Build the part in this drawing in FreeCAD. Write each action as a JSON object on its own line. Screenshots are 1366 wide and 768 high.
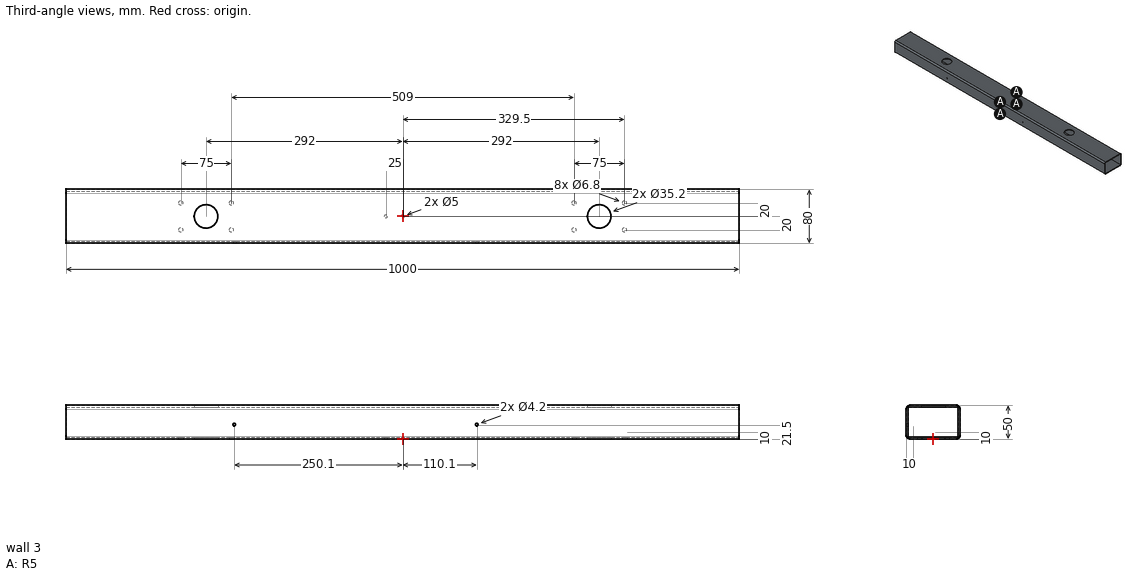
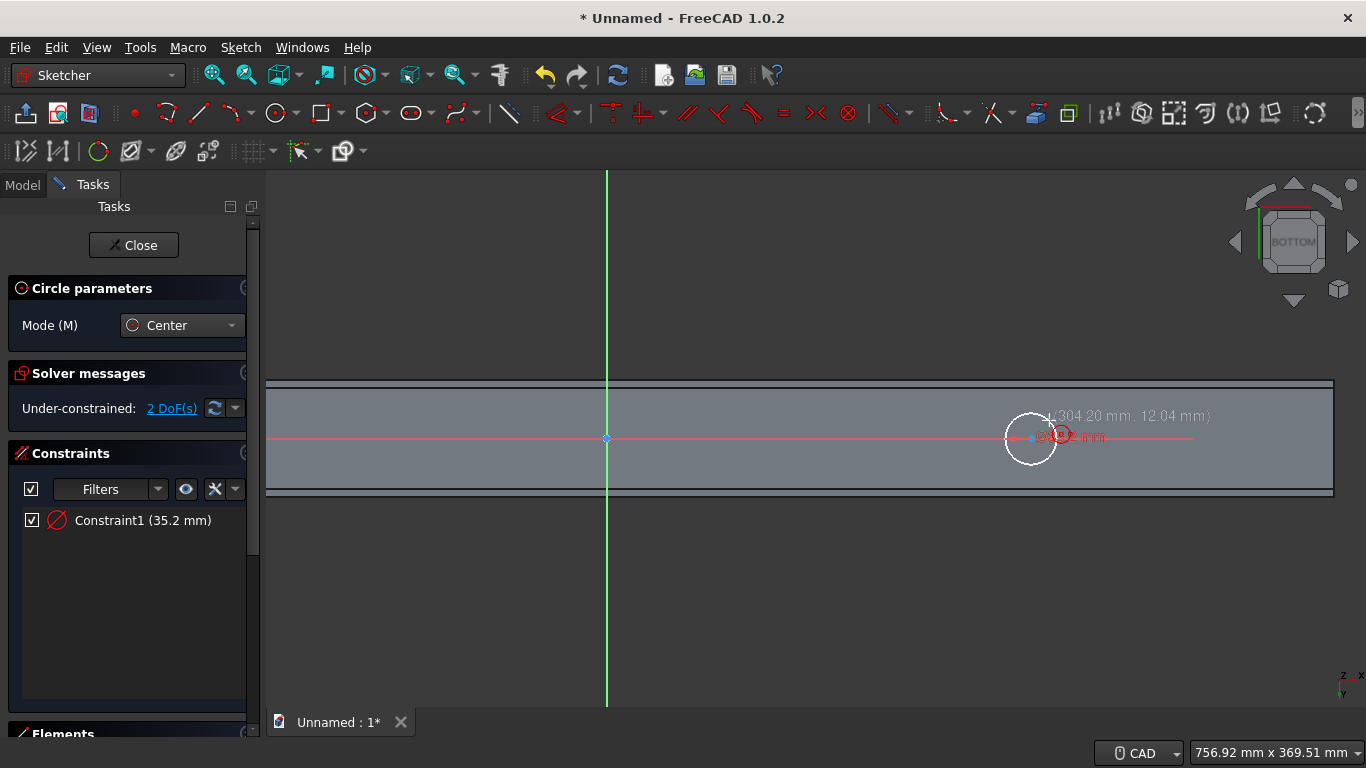
{"action": "scroll", "coordinate": [1033, 438], "scroll_direction": "down", "scroll_amount": 2}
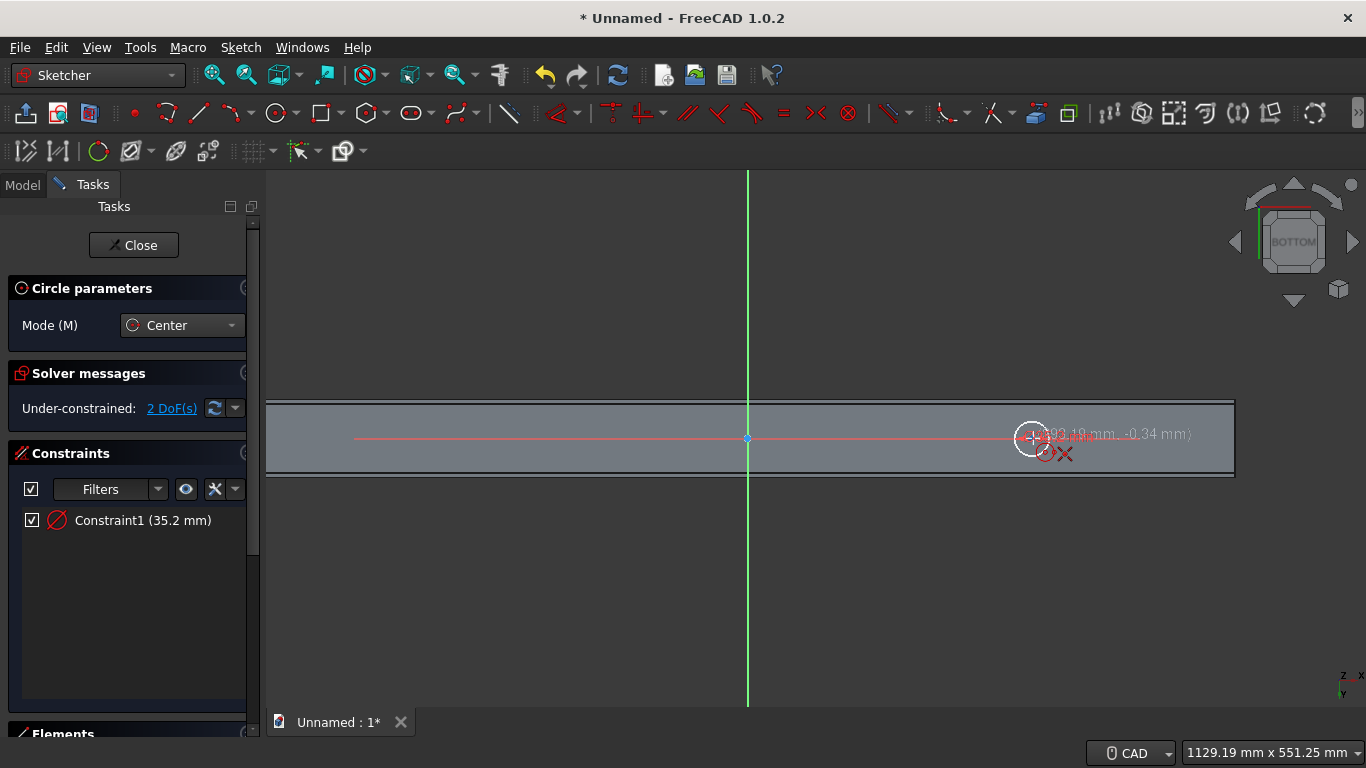
{"action": "scroll", "coordinate": [463, 438], "scroll_direction": "up", "scroll_amount": 2}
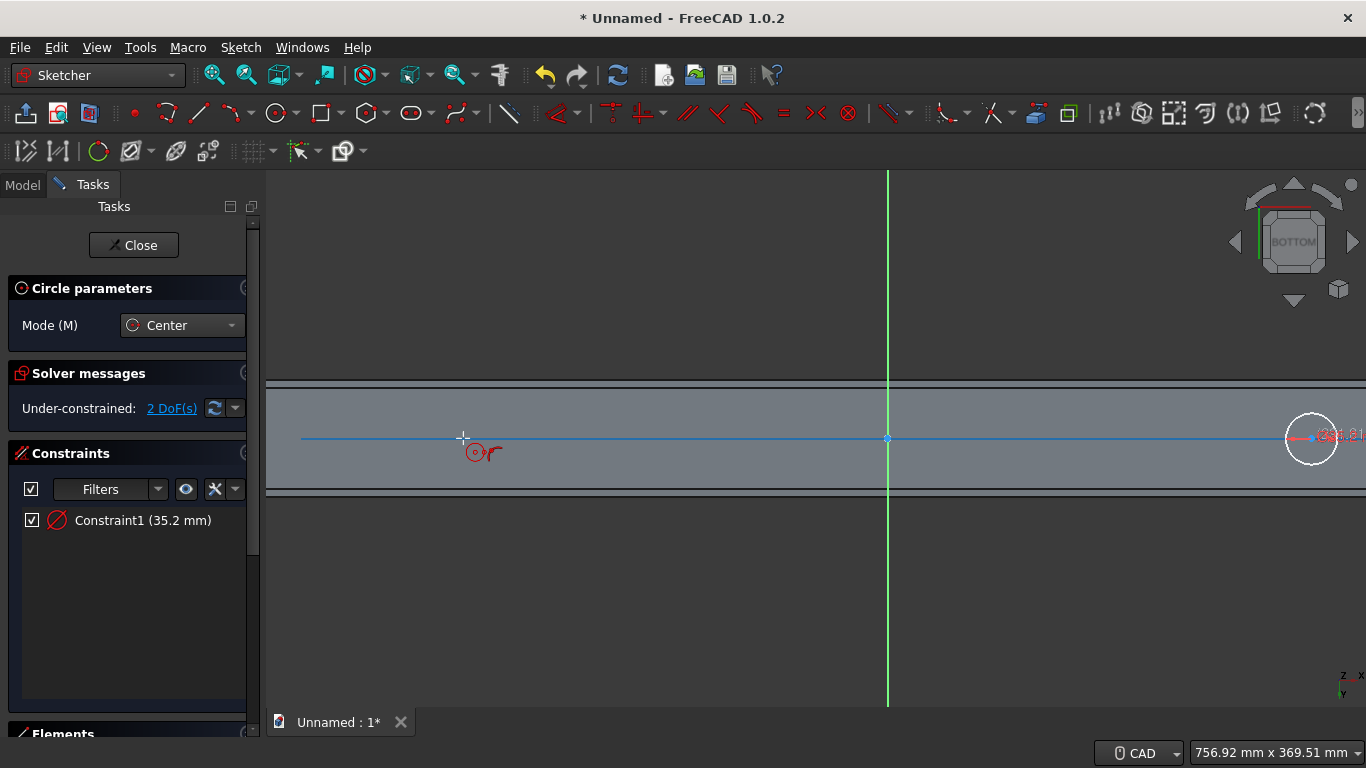
{"action": "left_click", "coordinate": [463, 438]}
{"action": "mouse_move", "coordinate": [481, 420]}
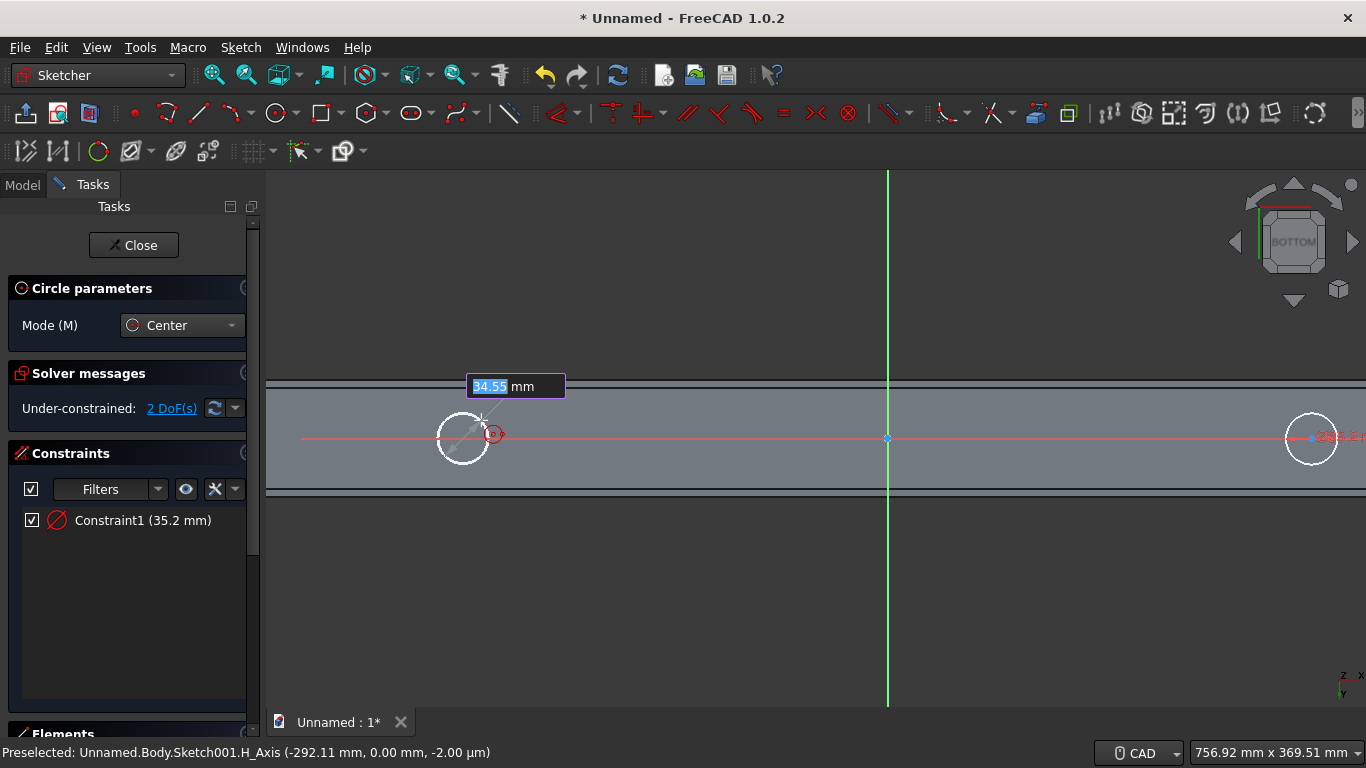
{"action": "type", "text": "35.2"}
{"action": "key", "text": "Return"}
{"action": "key", "text": "Escape"}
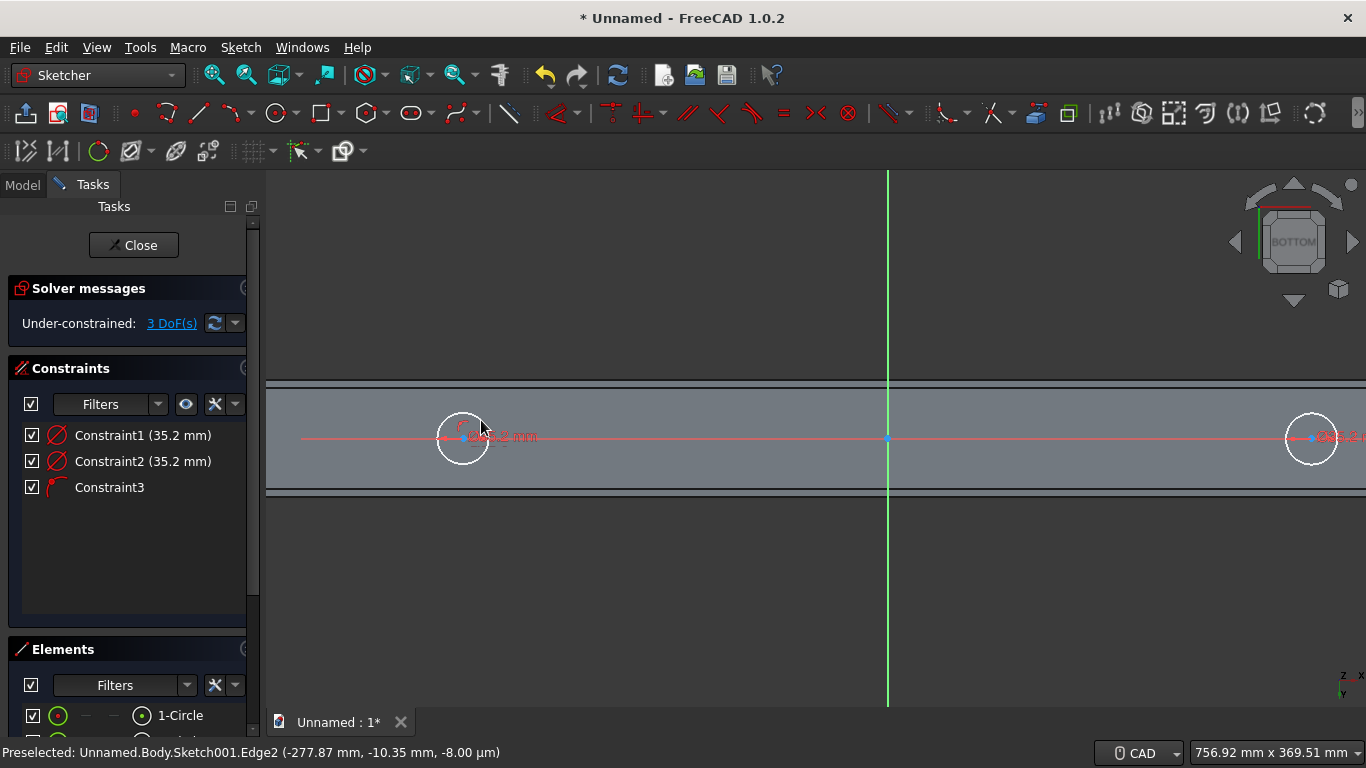
{"action": "scroll", "coordinate": [463, 438], "scroll_direction": "down", "scroll_amount": 2}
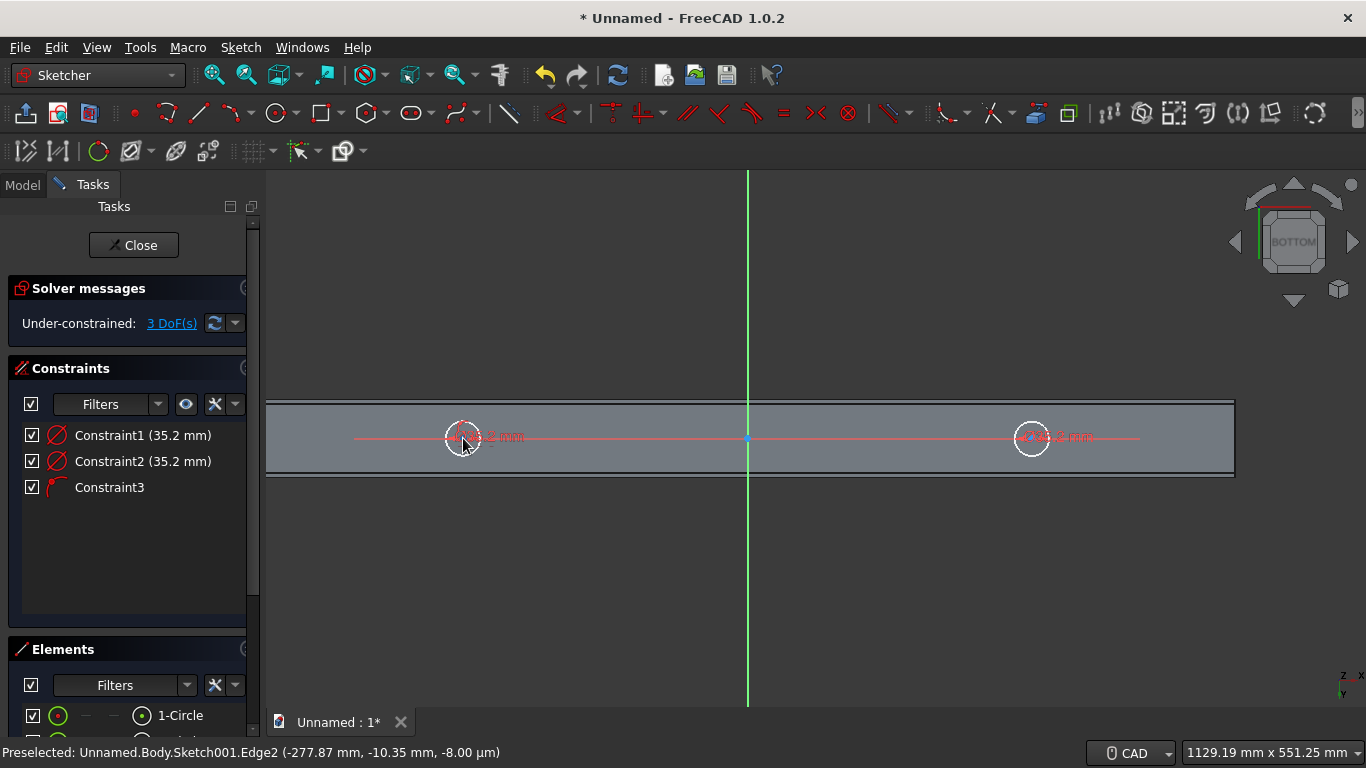
{"action": "left_click", "coordinate": [1032, 439]}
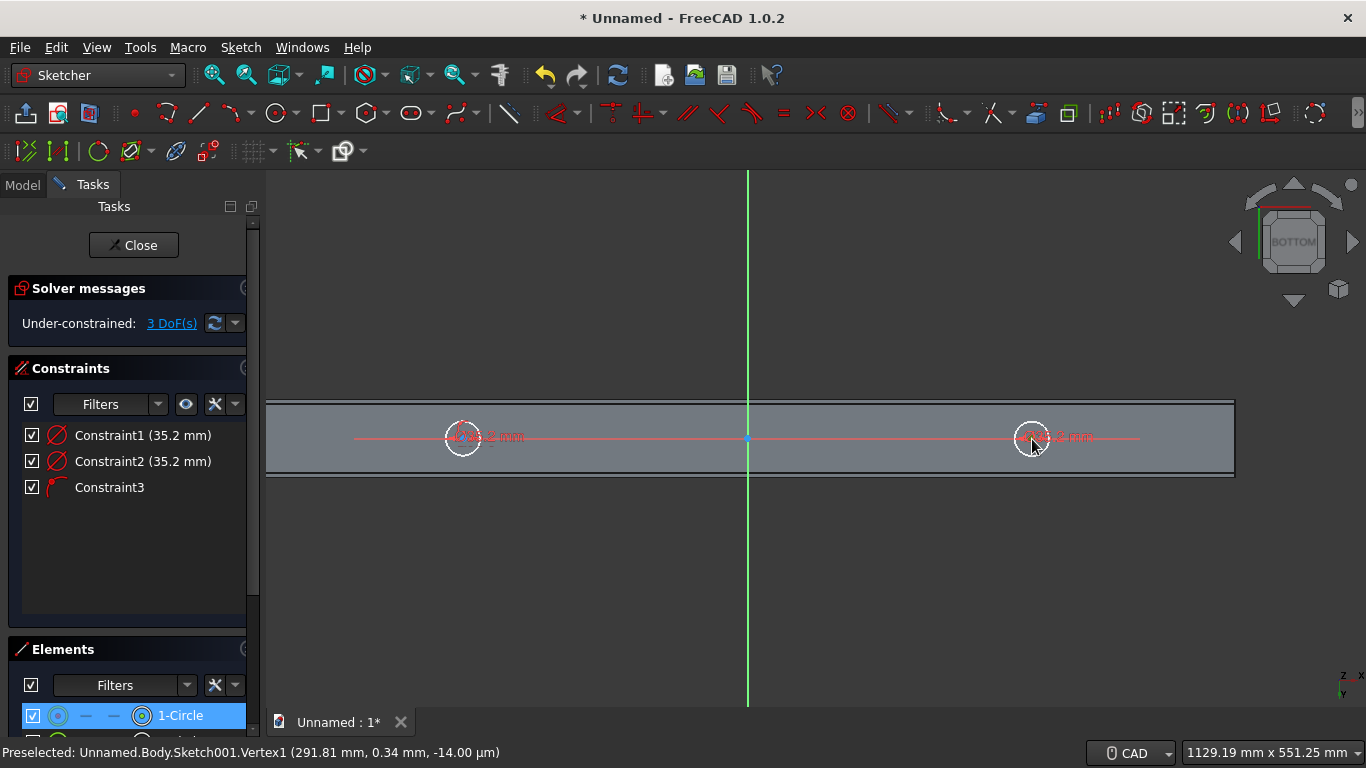
{"action": "left_click", "coordinate": [359, 438]}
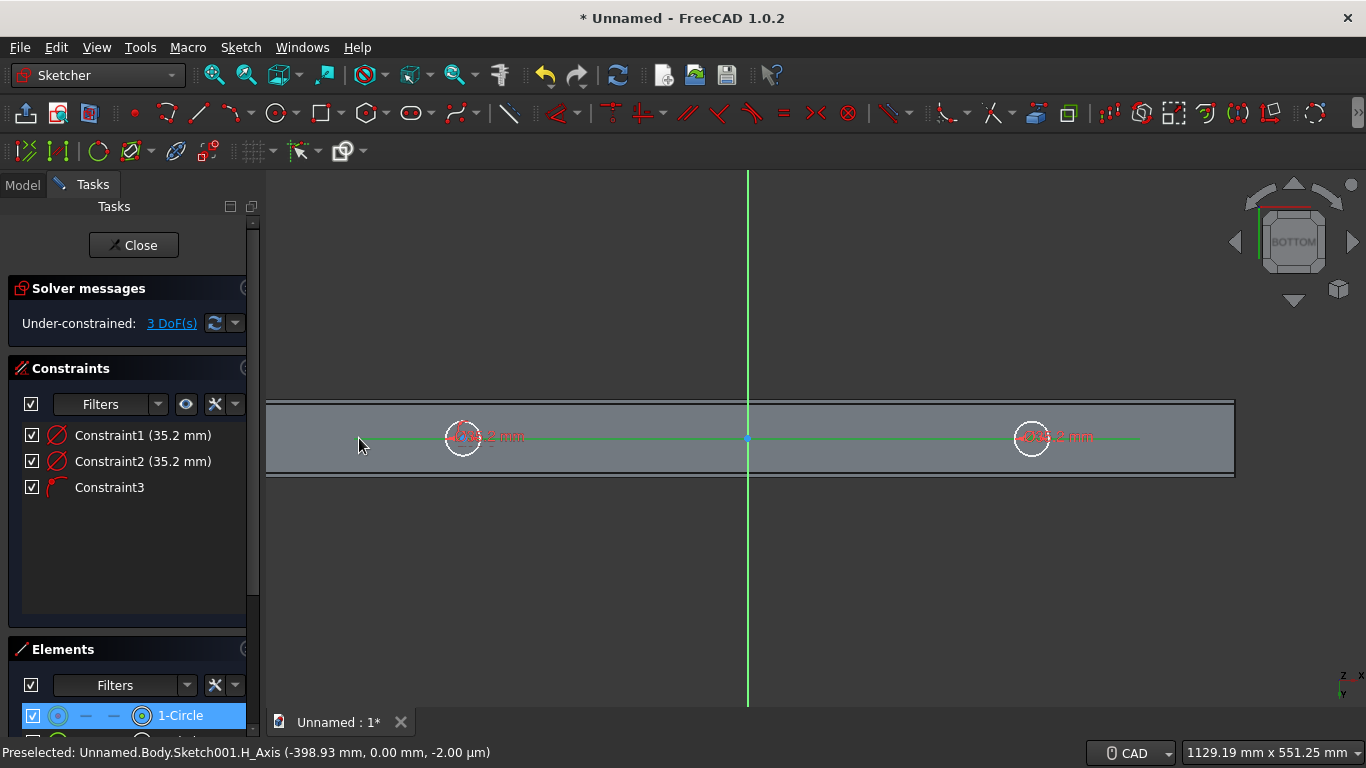
{"action": "key", "text": "c"}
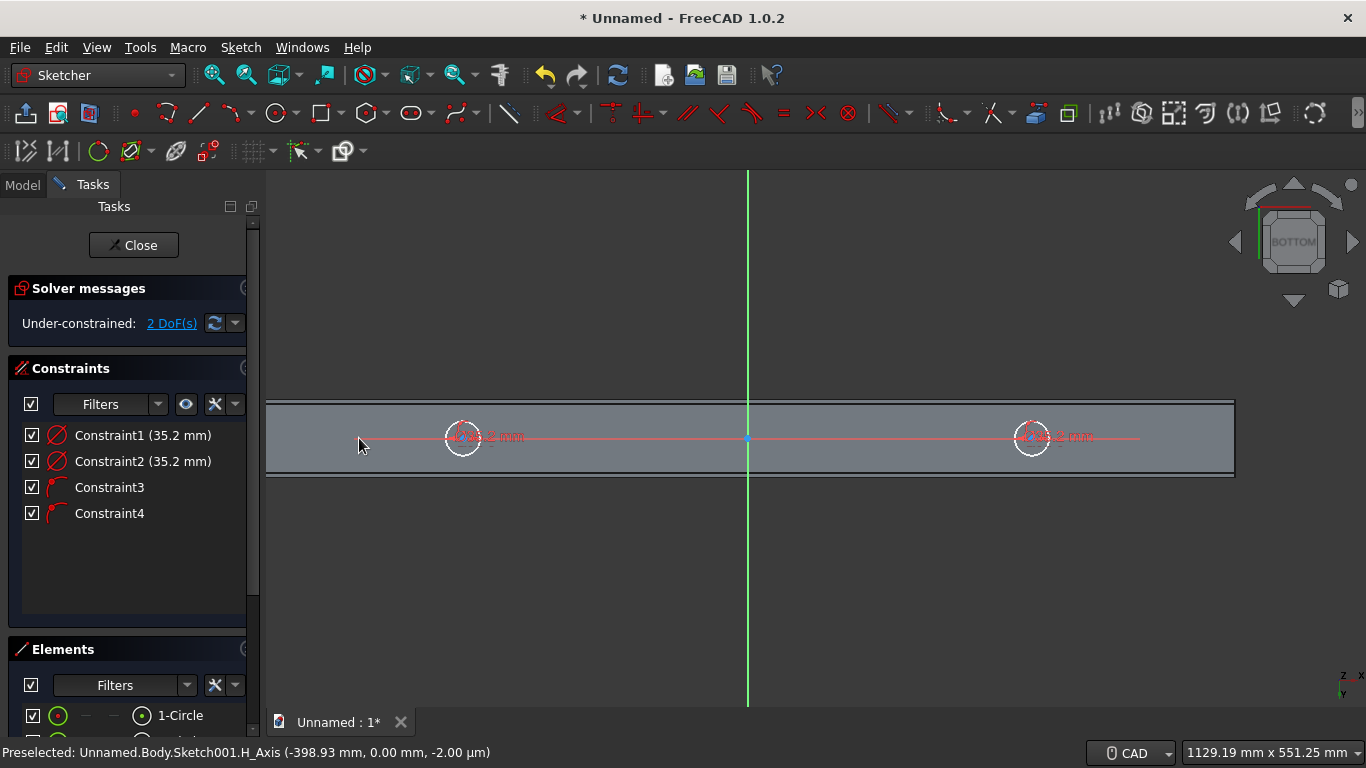
{"action": "left_click", "coordinate": [1032, 438]}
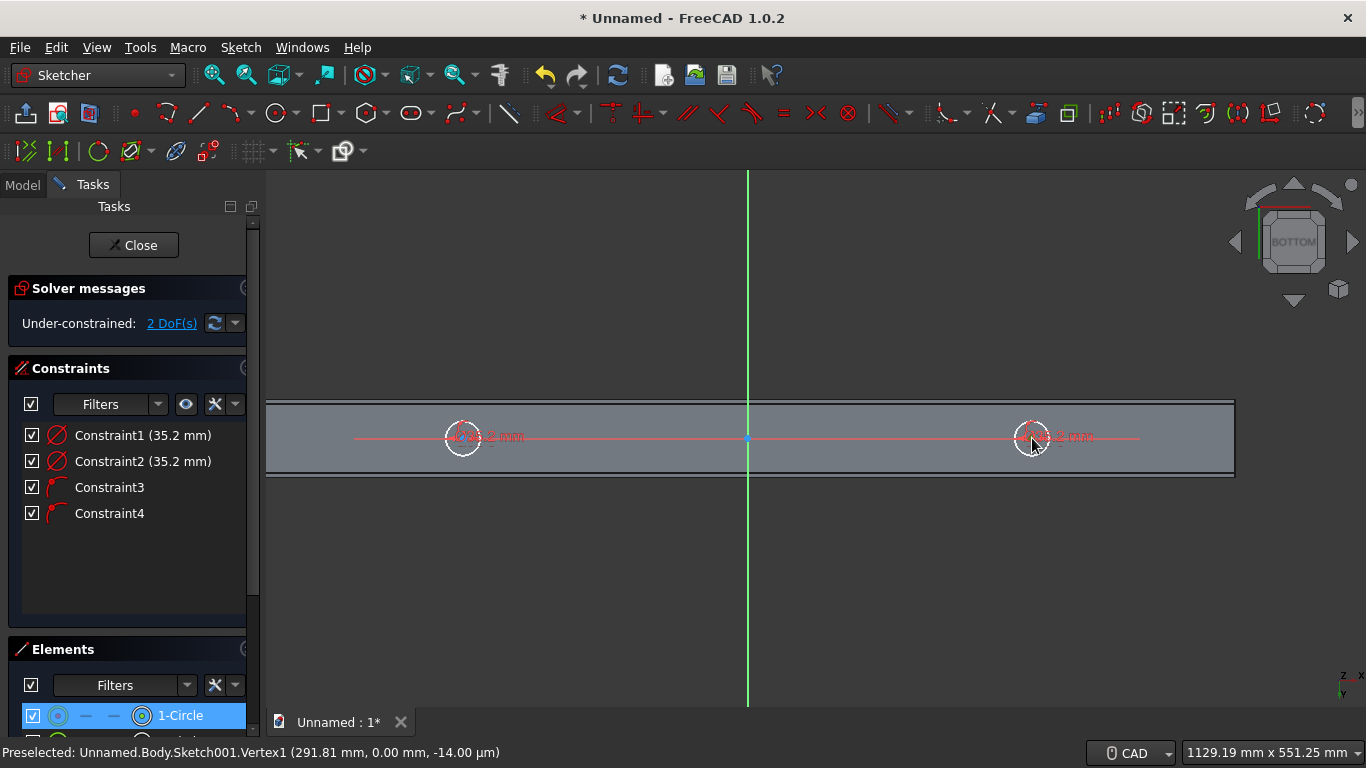
{"action": "key", "text": "l"}